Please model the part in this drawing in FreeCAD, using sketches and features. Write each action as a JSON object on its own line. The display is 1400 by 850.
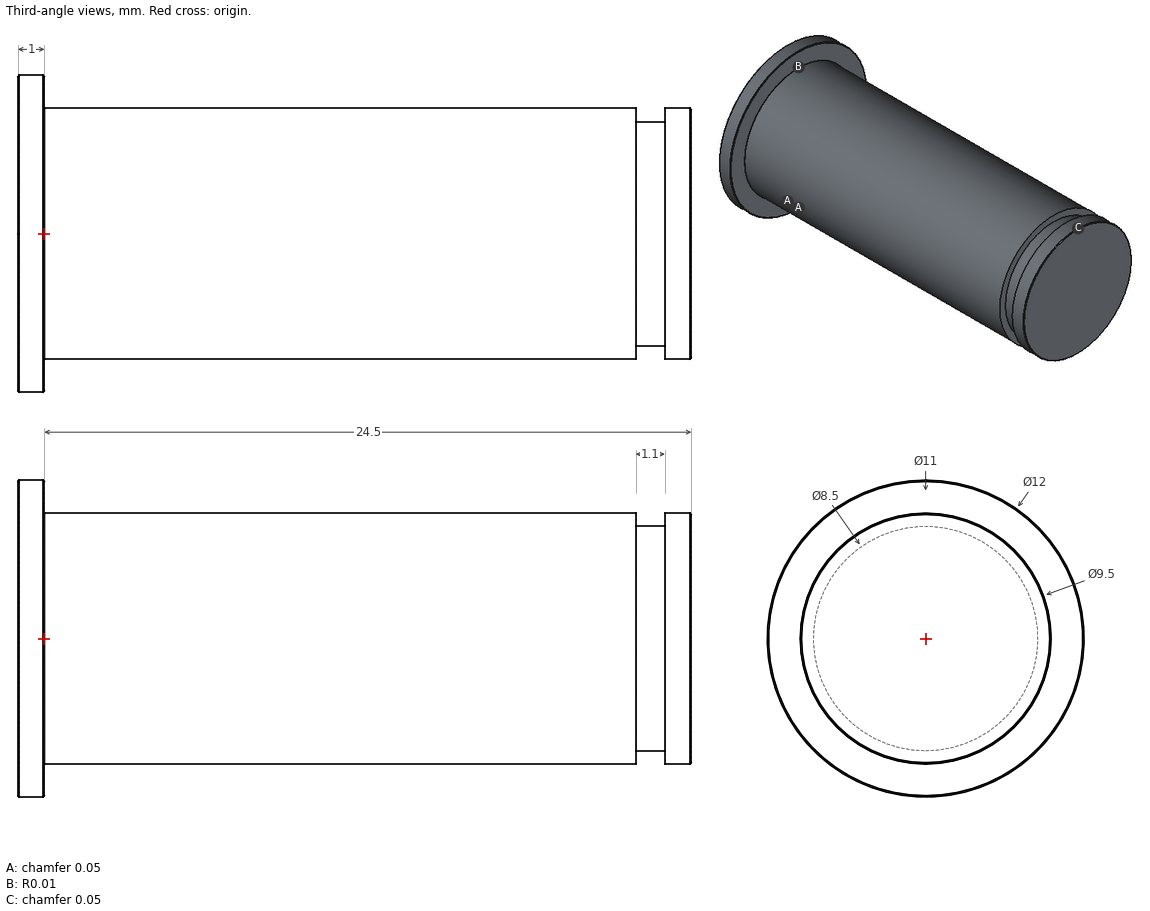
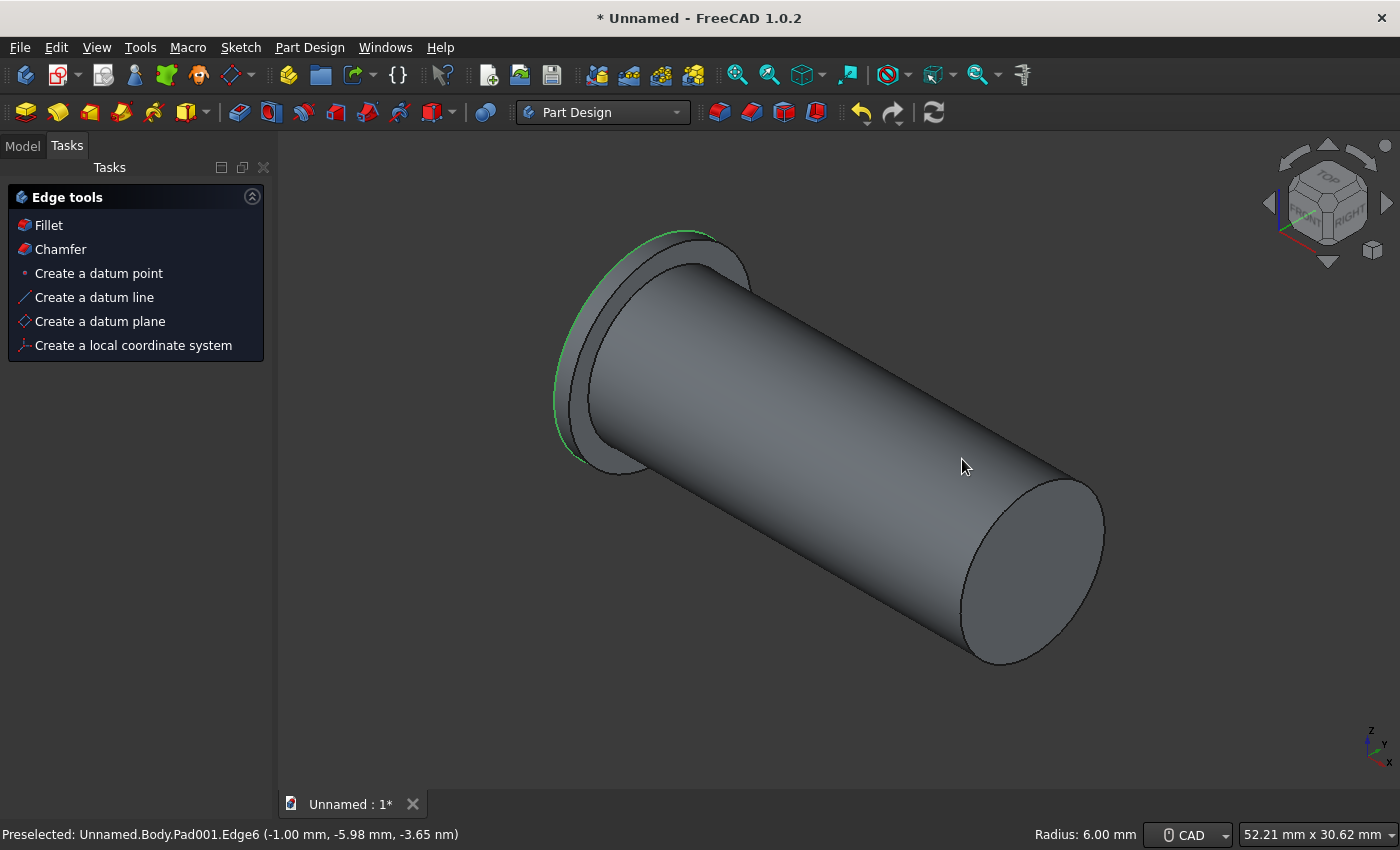
{"action": "left_click", "coordinate": [569, 409], "text": "ctrl"}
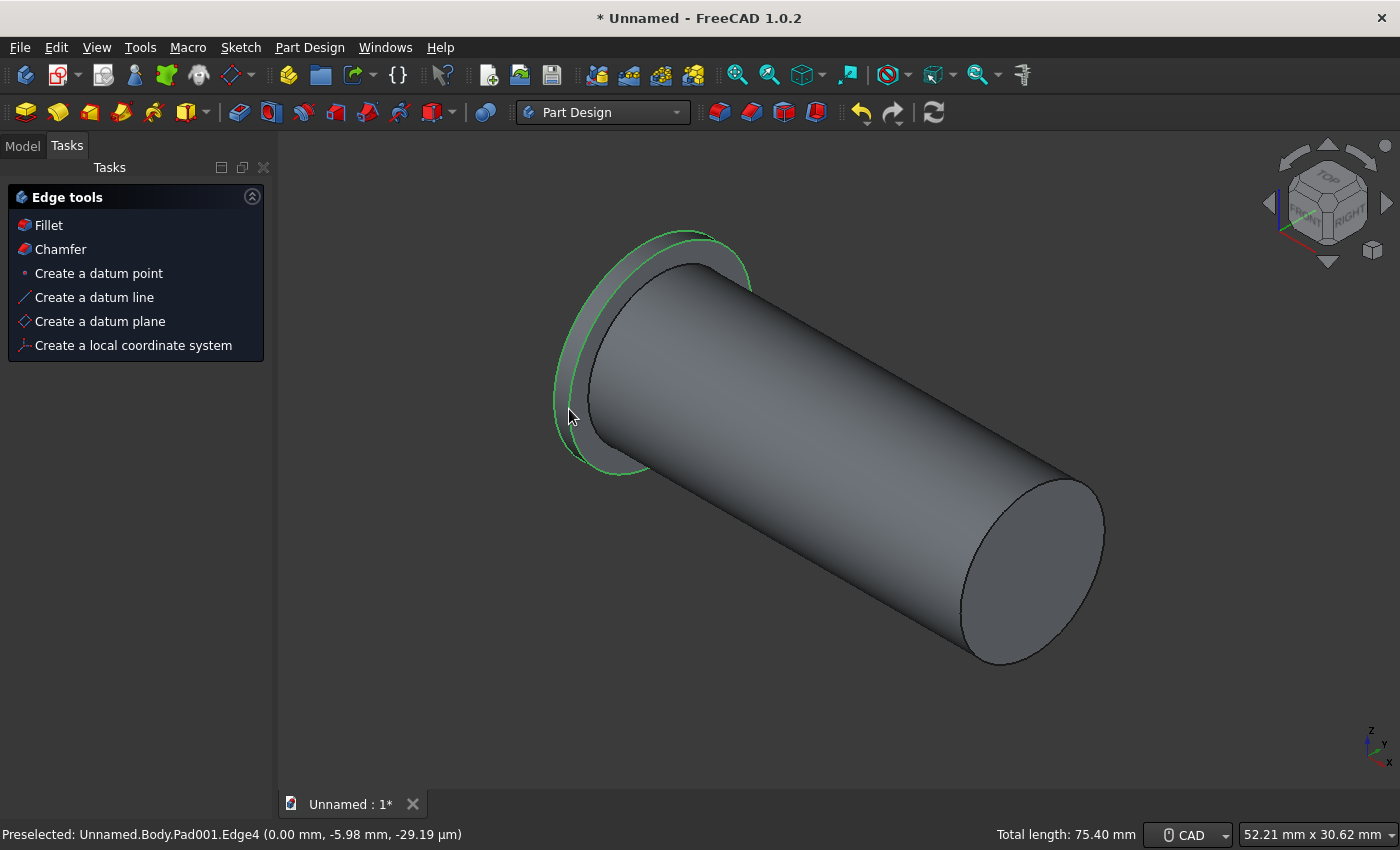
{"action": "left_click", "coordinate": [752, 112]}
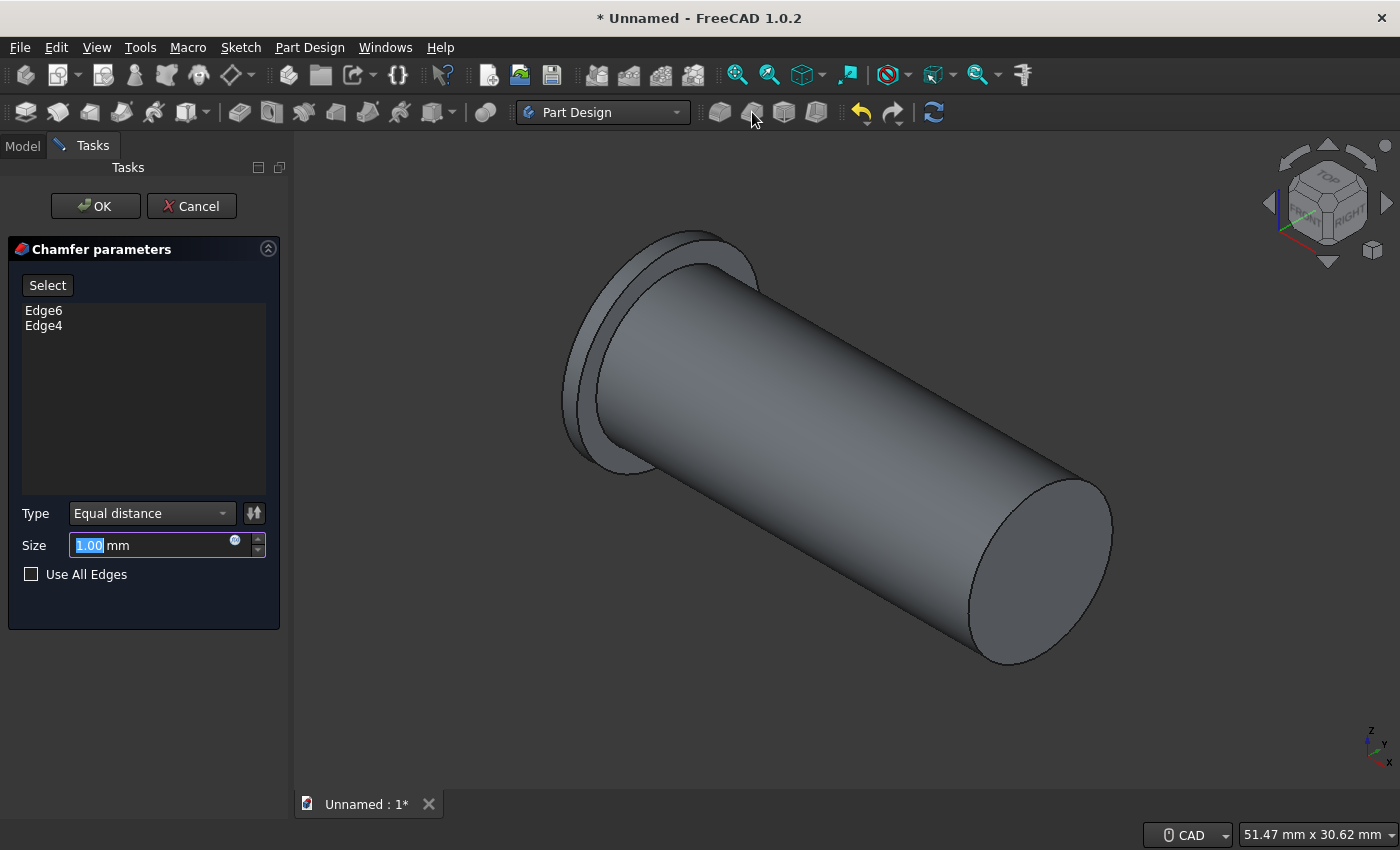
{"action": "type", "text": "0.05"}
{"action": "key", "text": "Tab"}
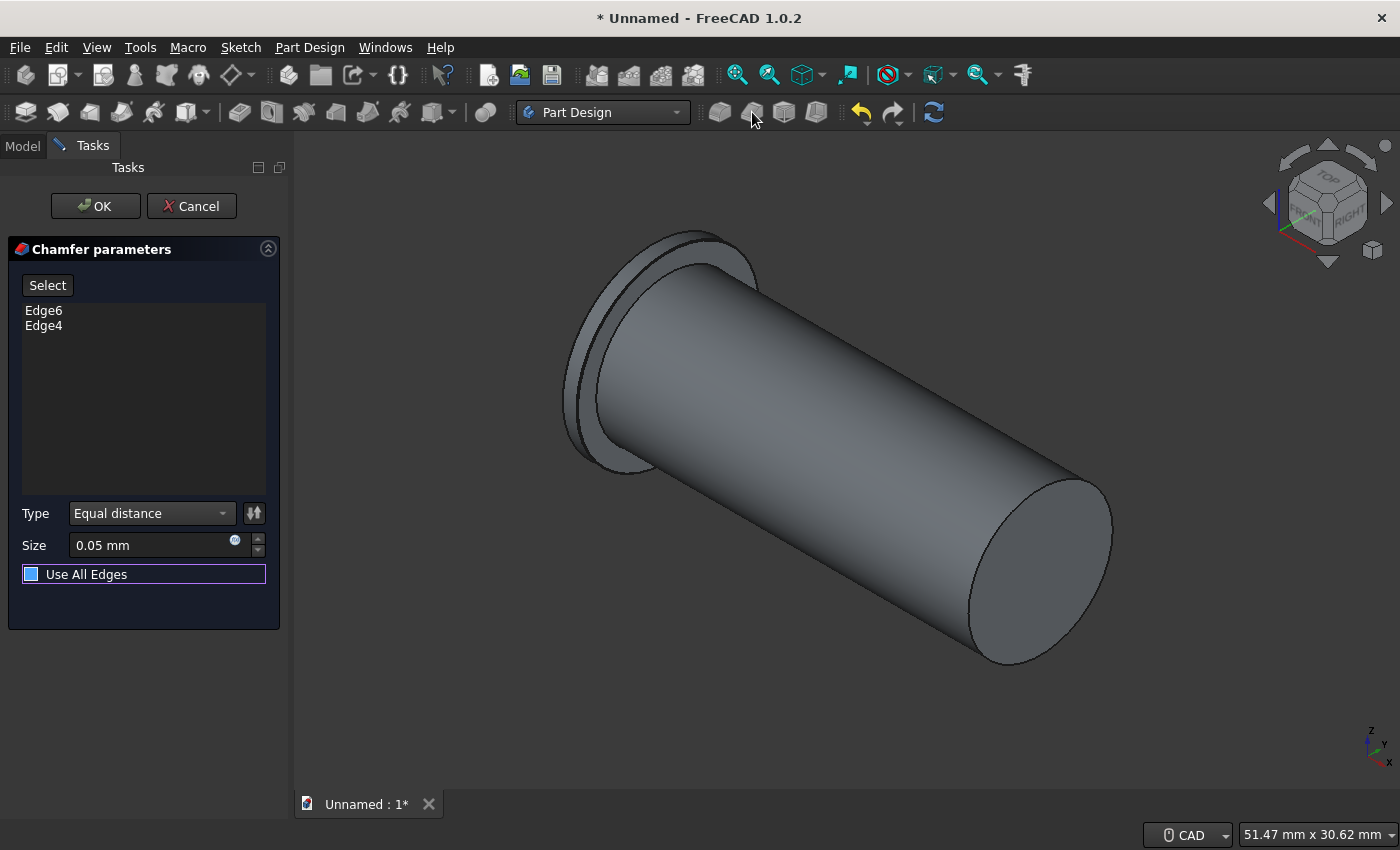
{"action": "left_click", "coordinate": [96, 206]}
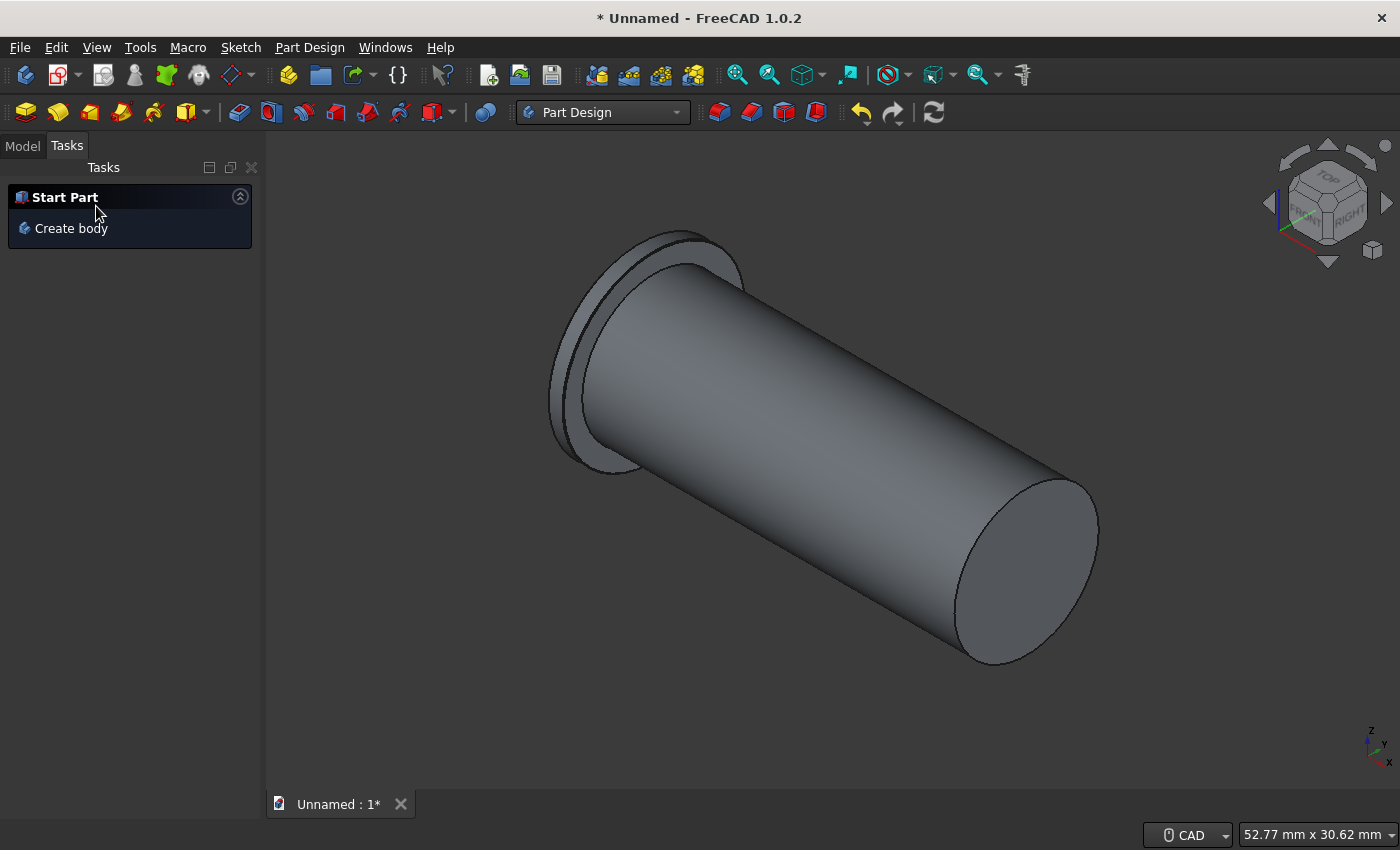
{"action": "key", "text": "2"}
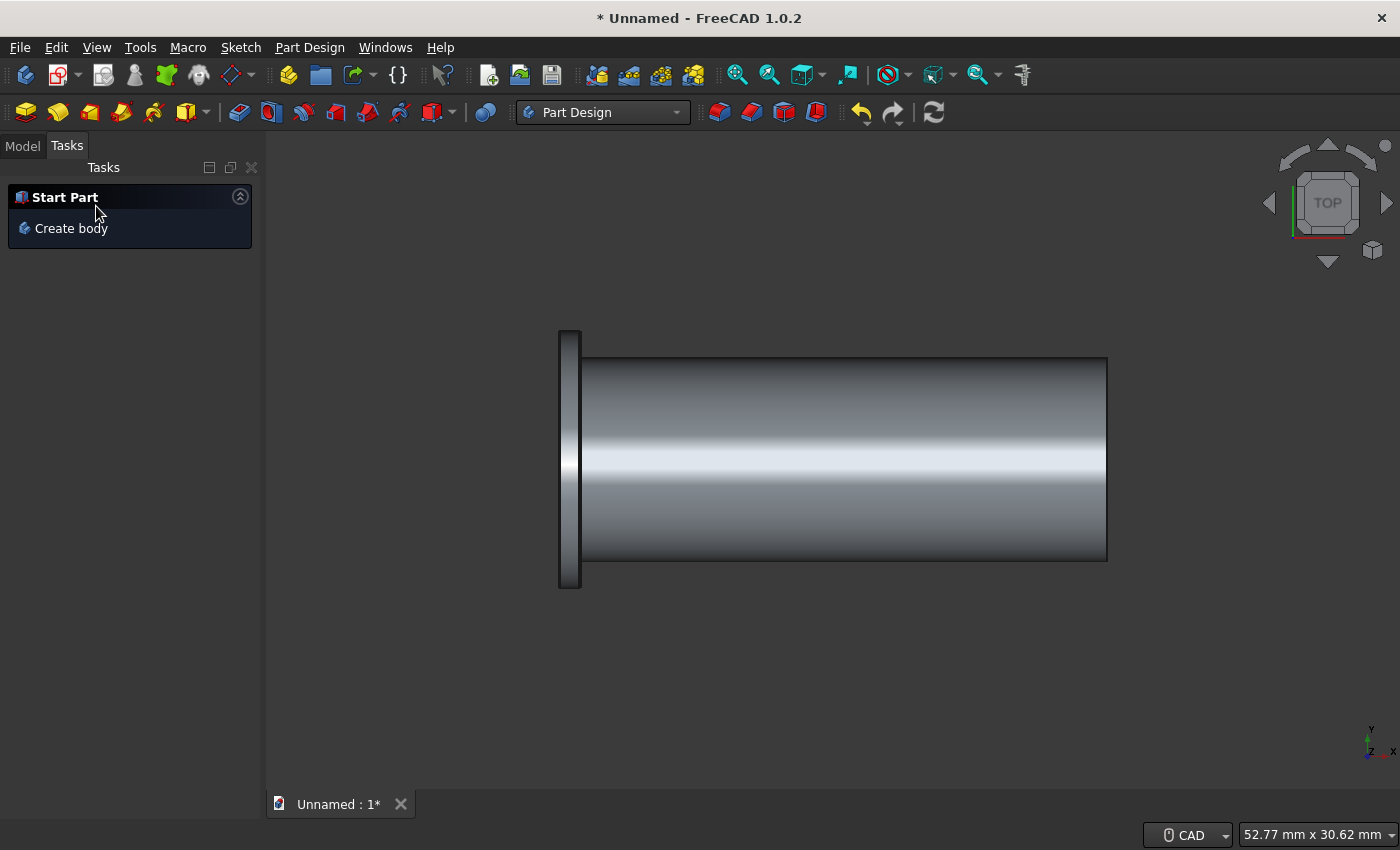
{"action": "key", "text": "0"}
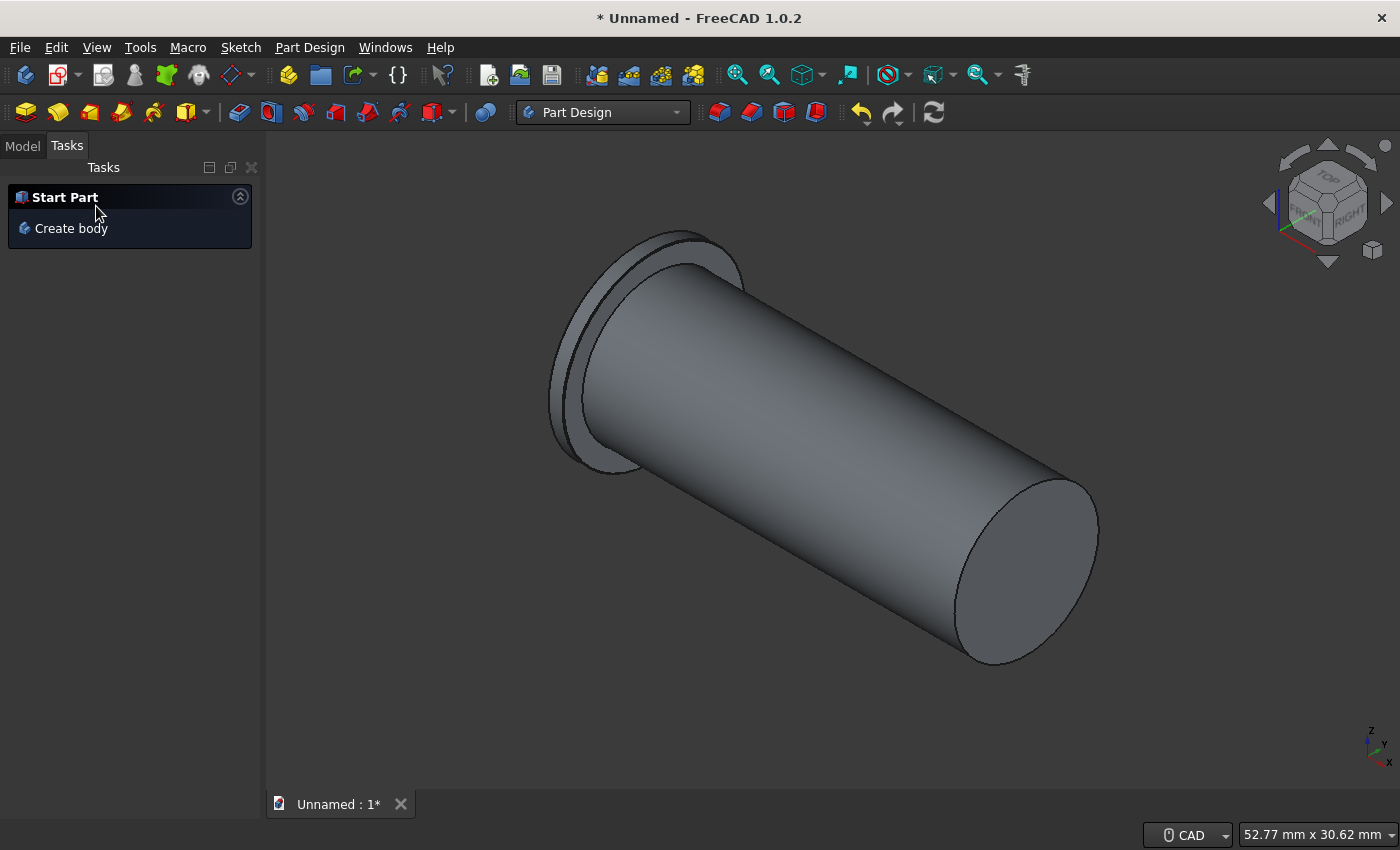
{"action": "key", "text": "1"}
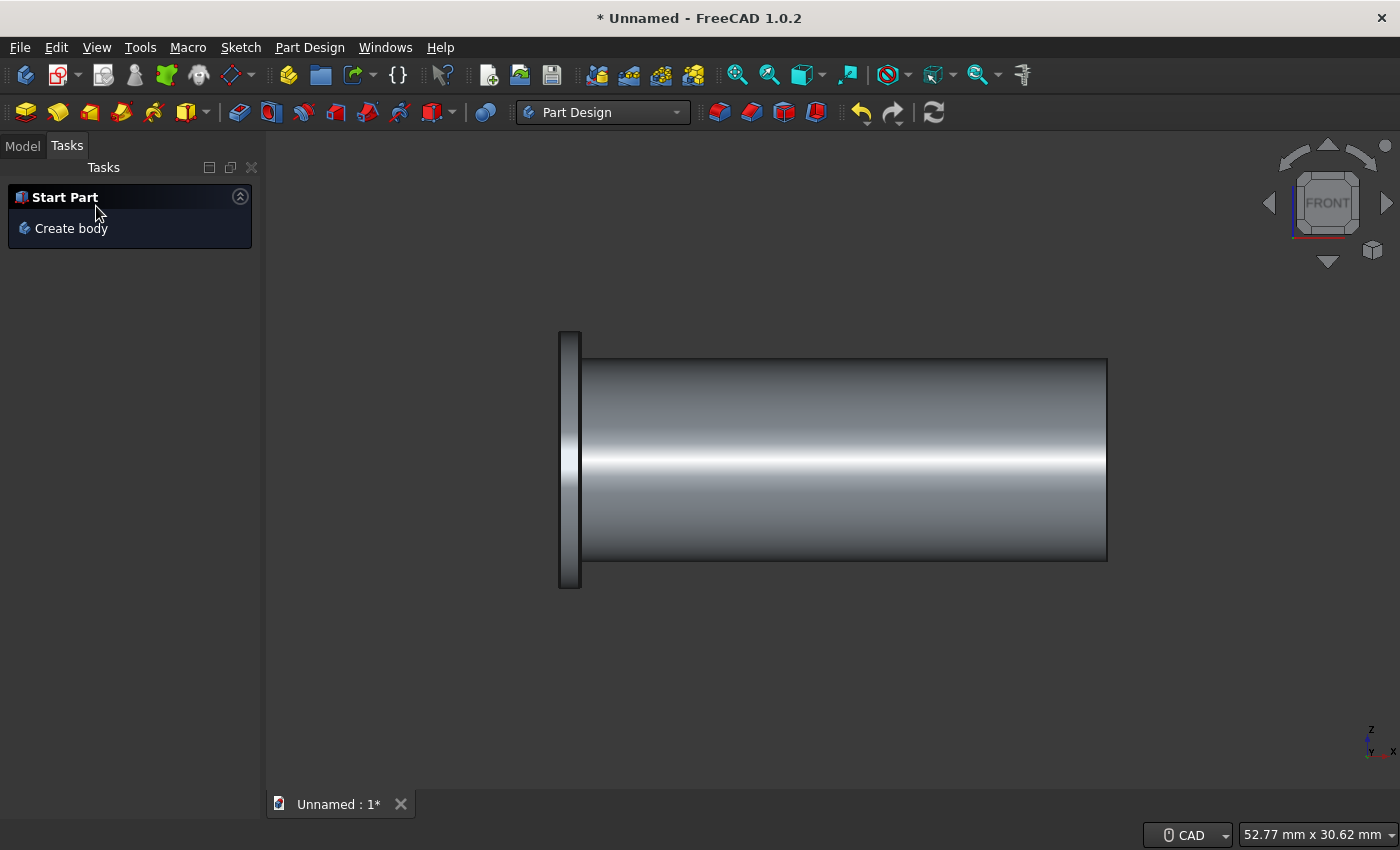
{"action": "key", "text": "3"}